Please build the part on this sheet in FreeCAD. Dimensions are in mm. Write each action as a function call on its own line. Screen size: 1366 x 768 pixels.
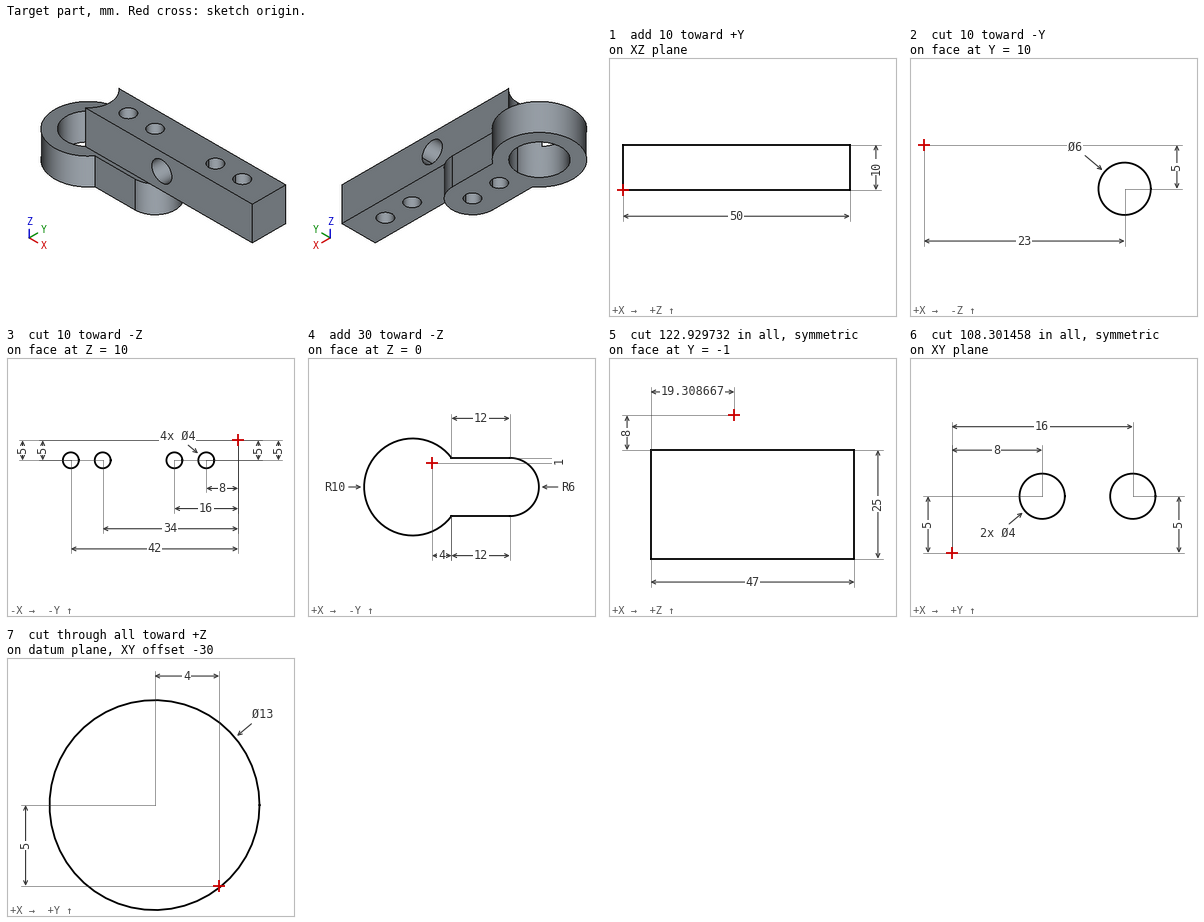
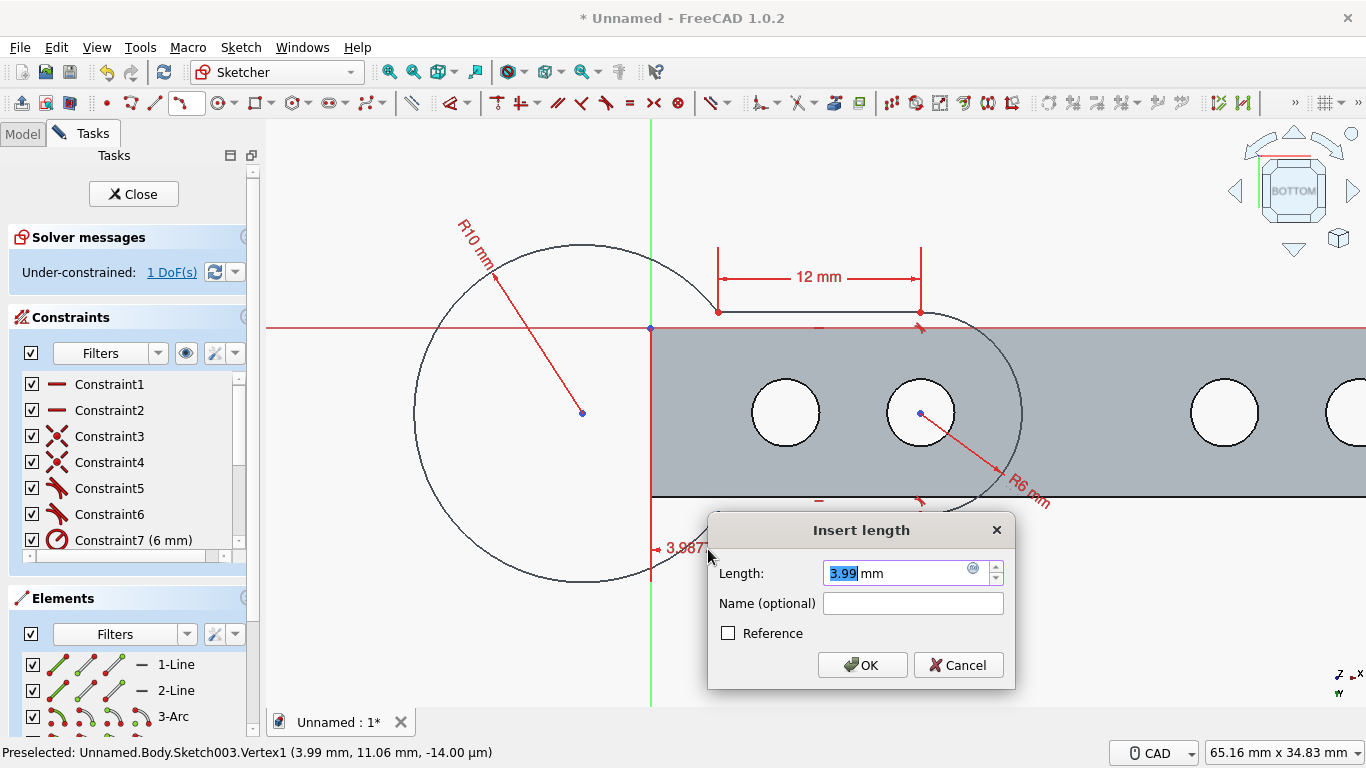
text(4)
key(Return)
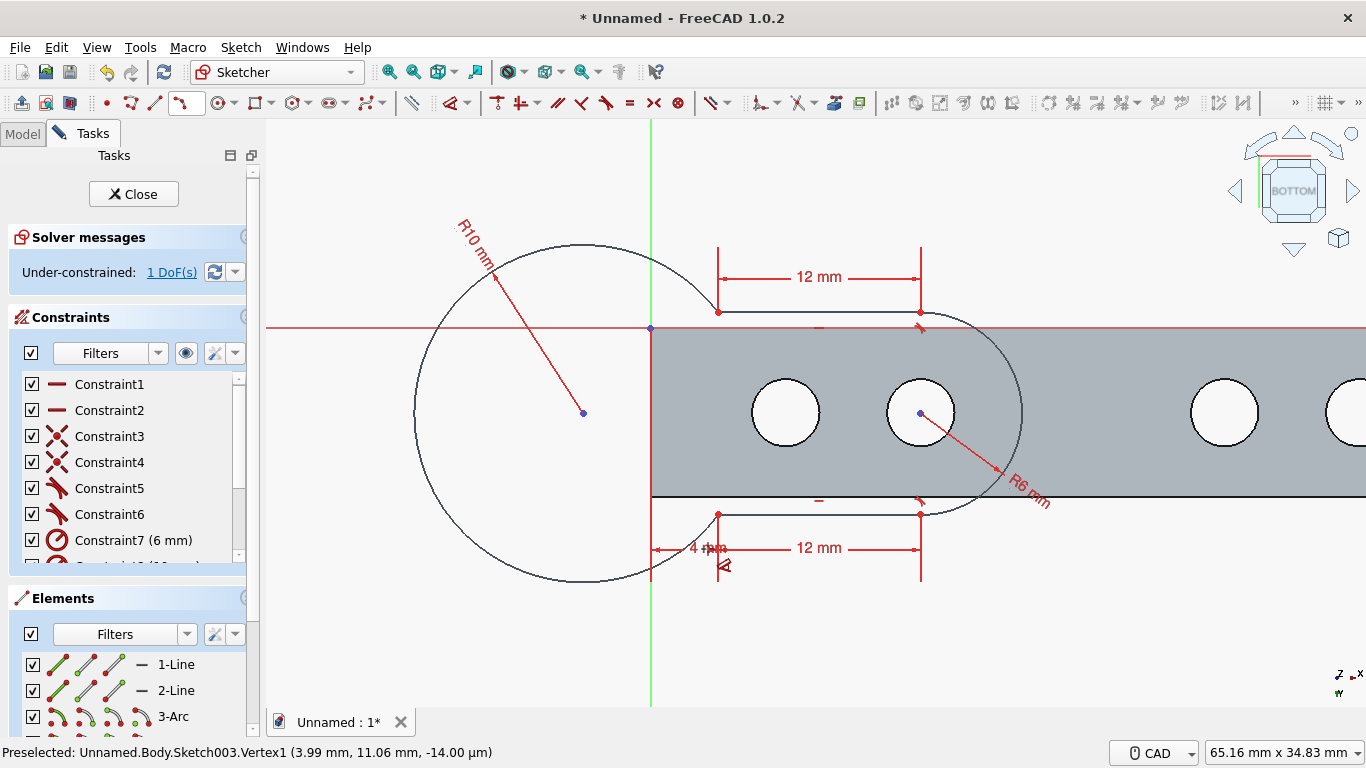
scroll(921, 312, up, 5)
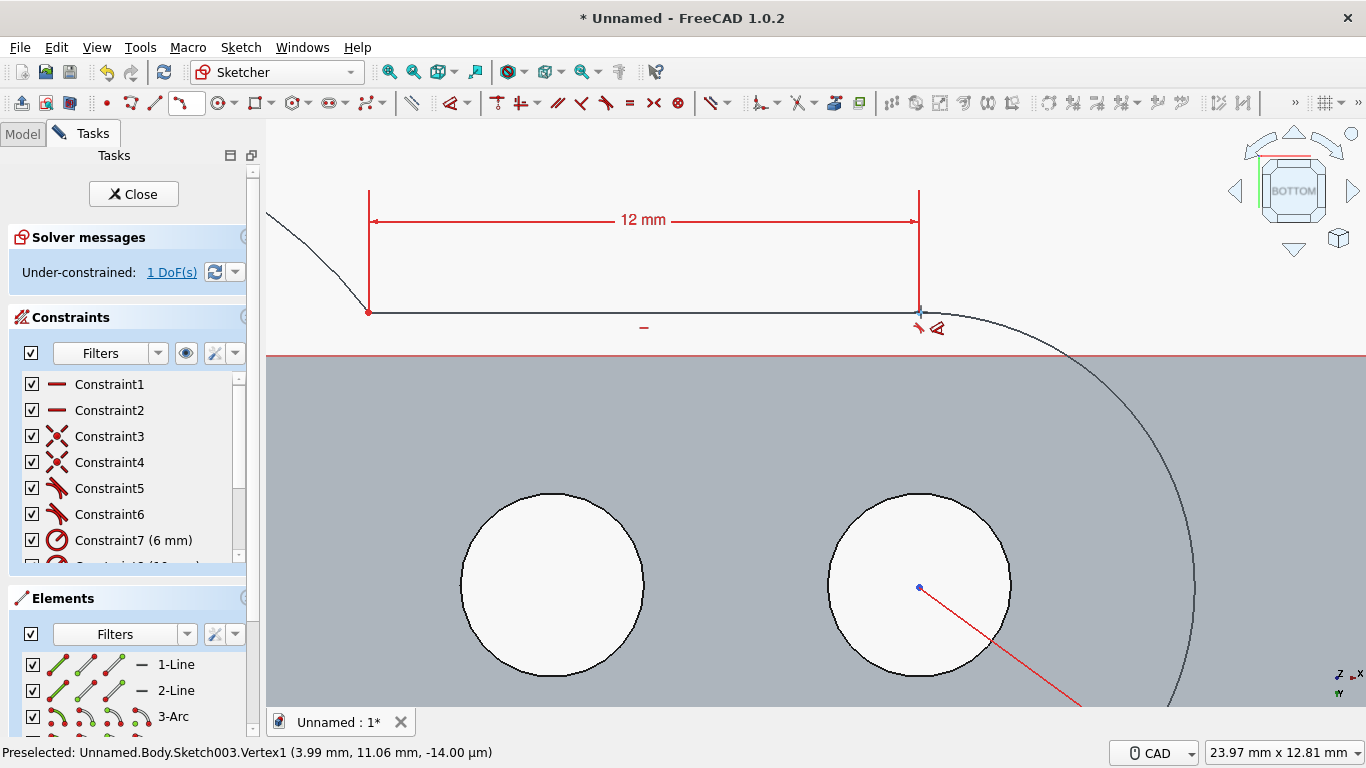
click(919, 313)
click(953, 334)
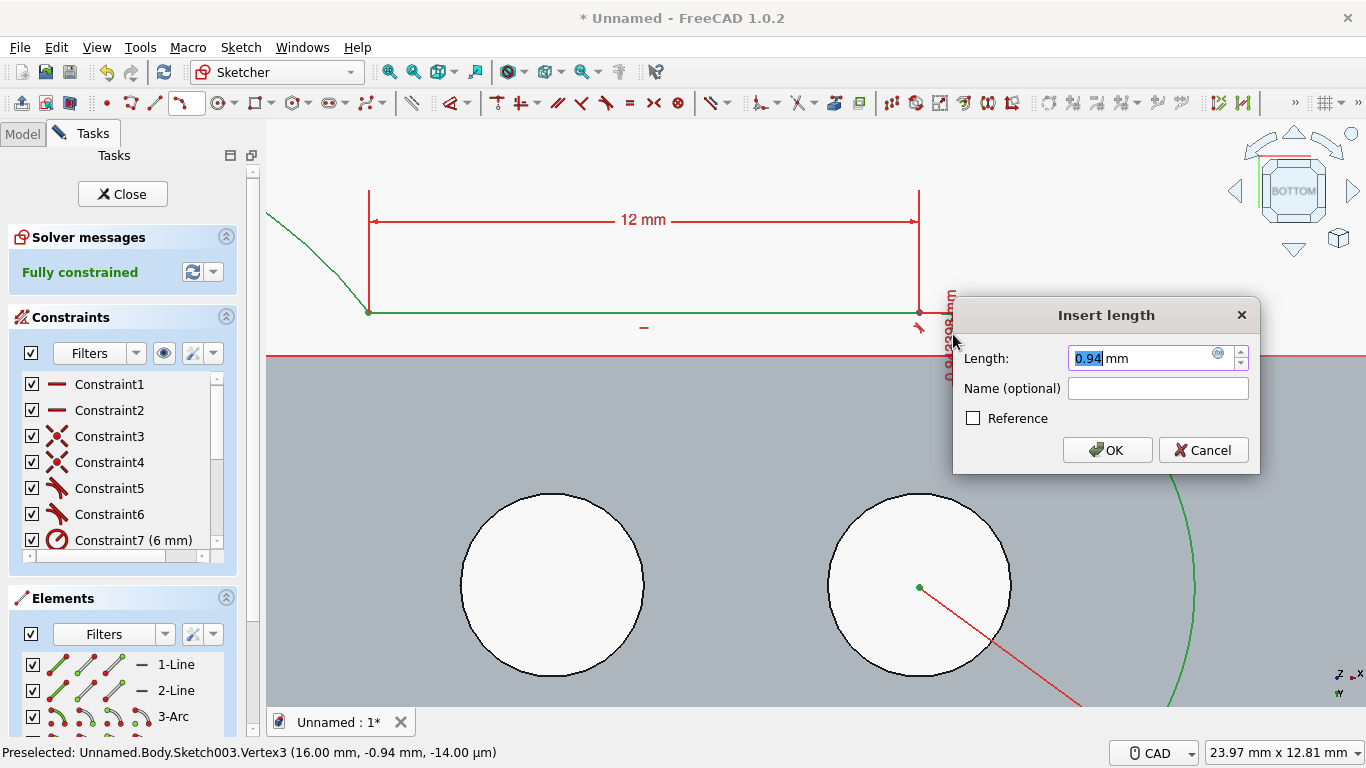
text(1)
key(Return)
key(Escape)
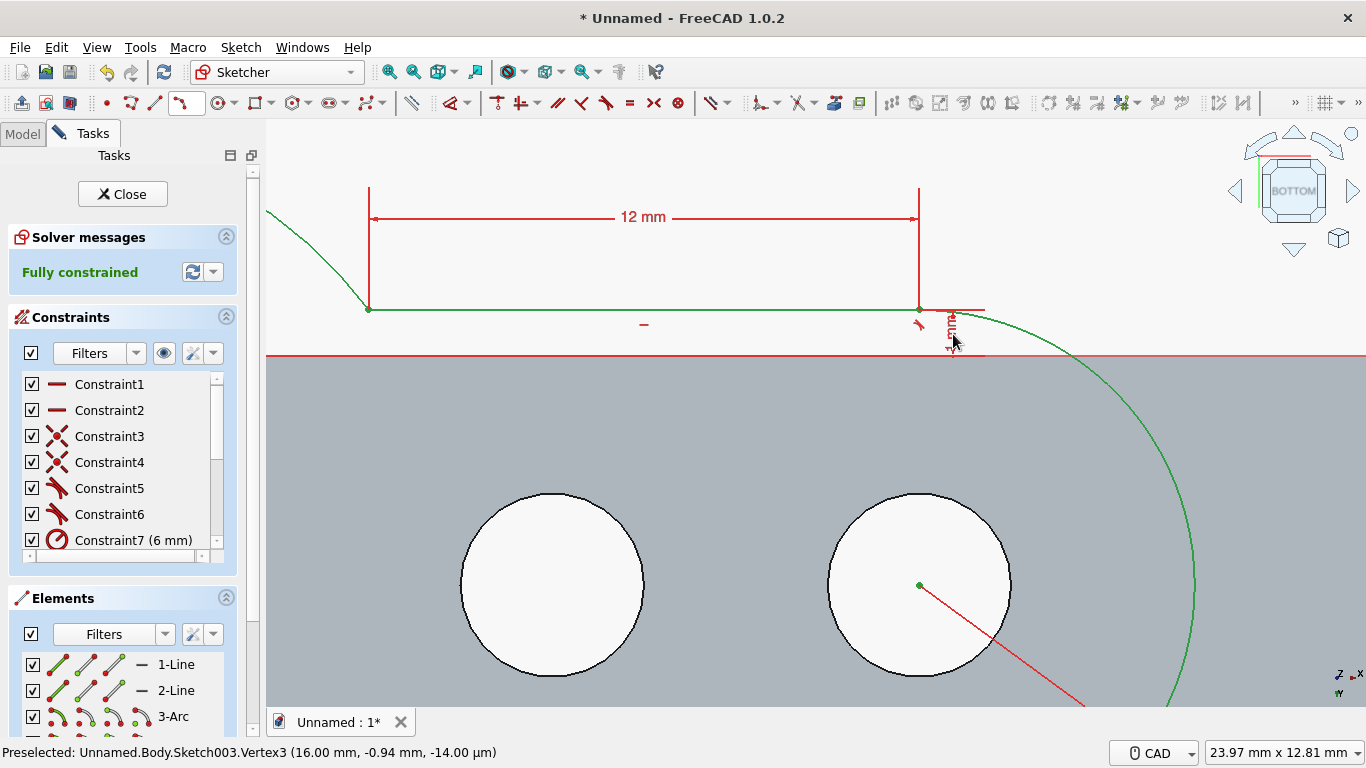
click(123, 194)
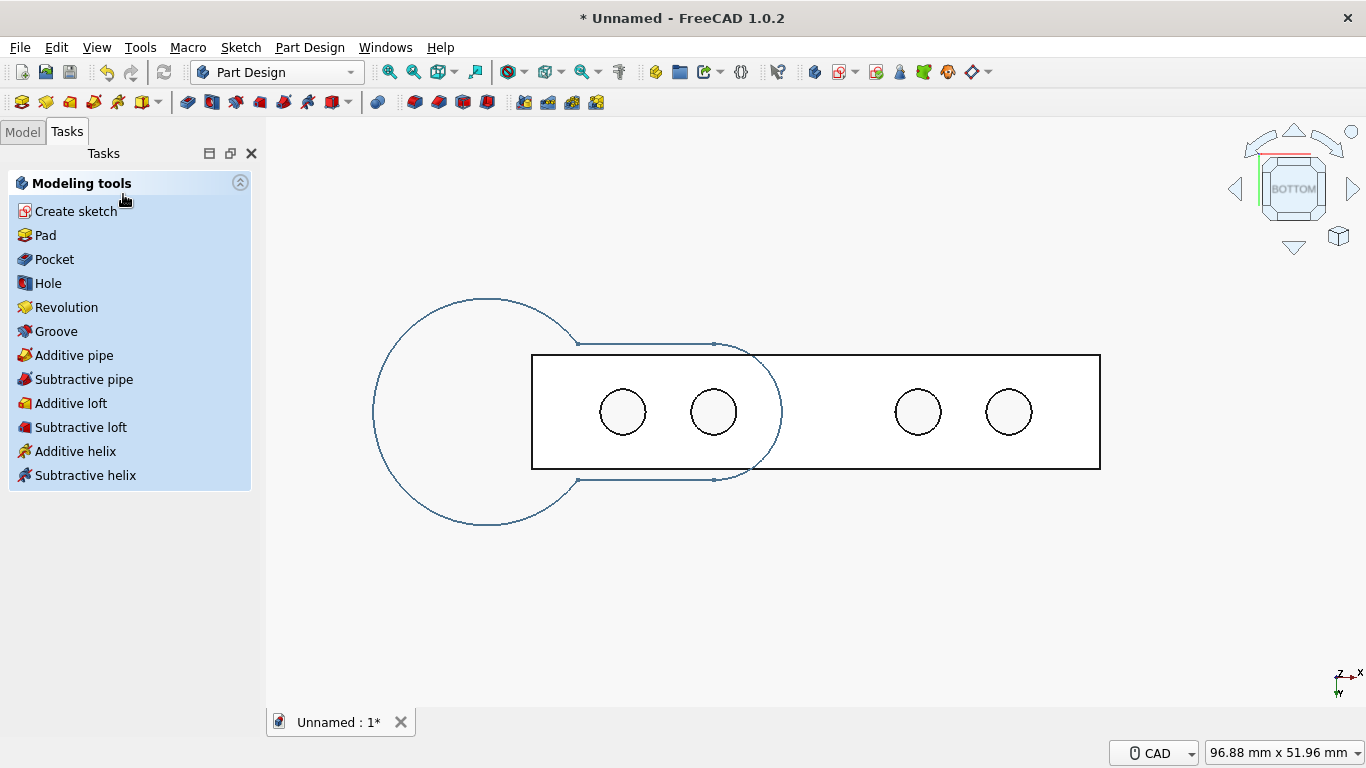
click(22, 102)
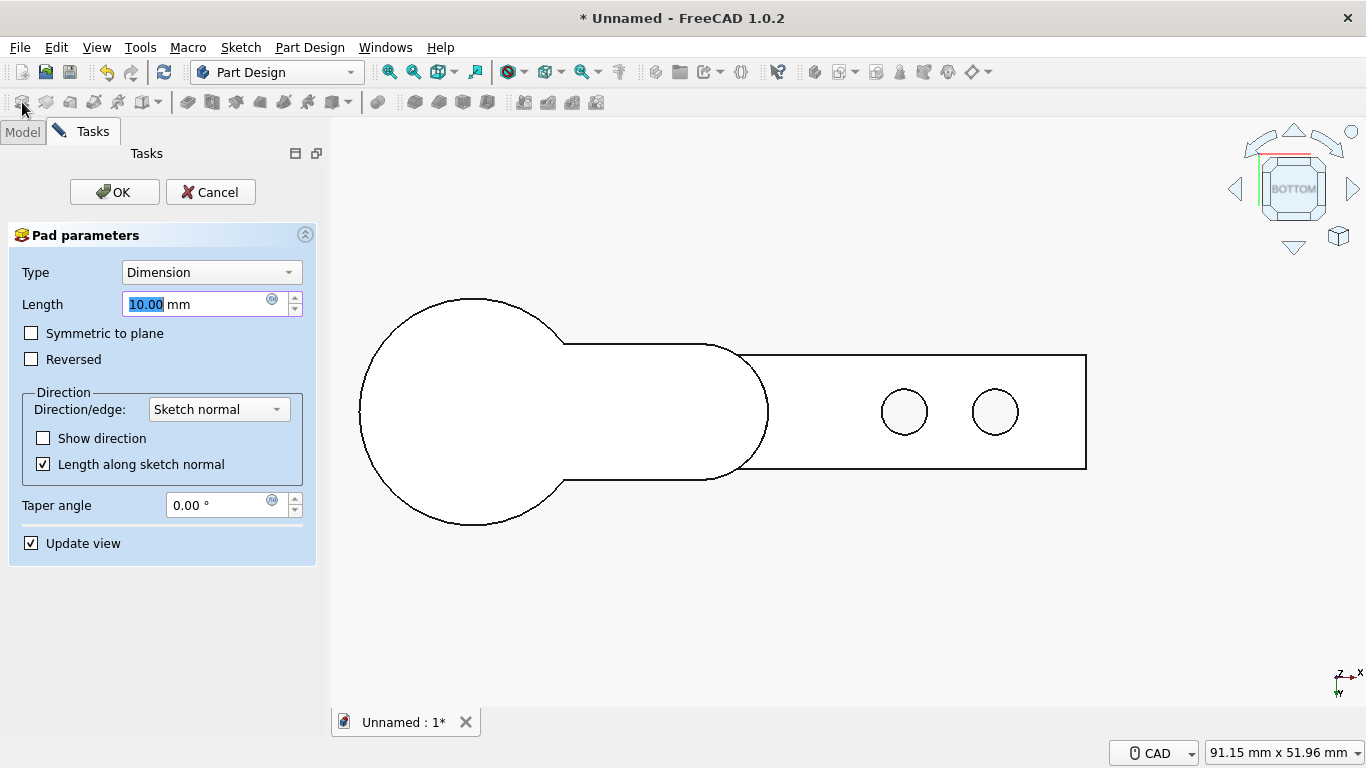
text(30)
key(Tab)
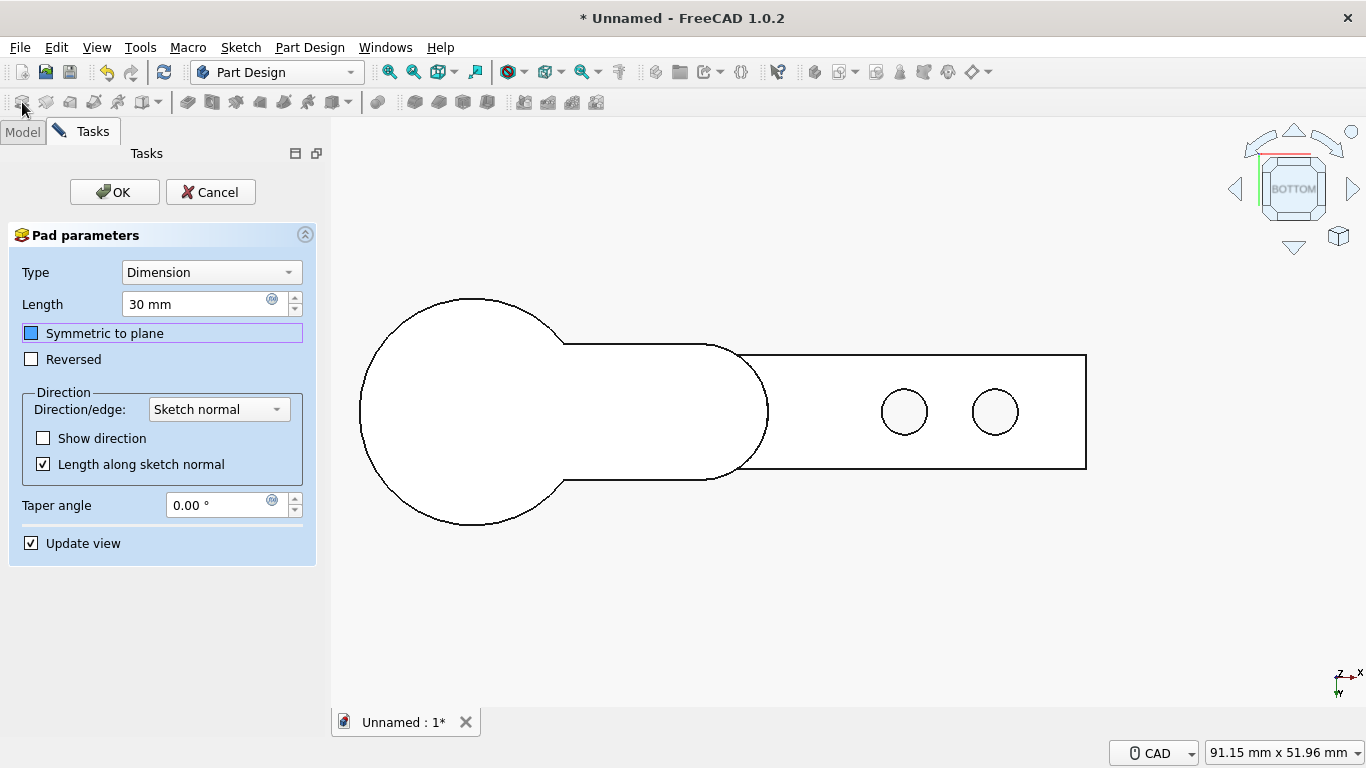
click(115, 192)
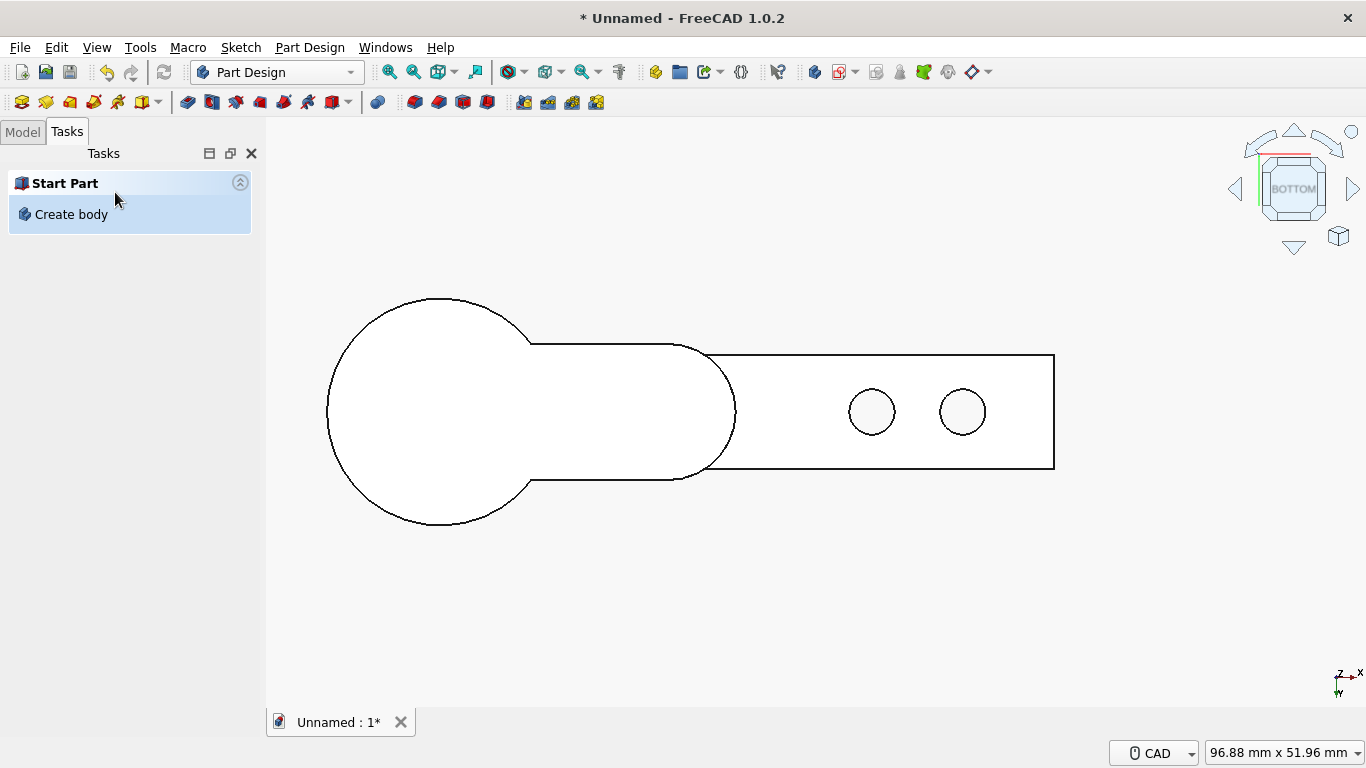
key(0)